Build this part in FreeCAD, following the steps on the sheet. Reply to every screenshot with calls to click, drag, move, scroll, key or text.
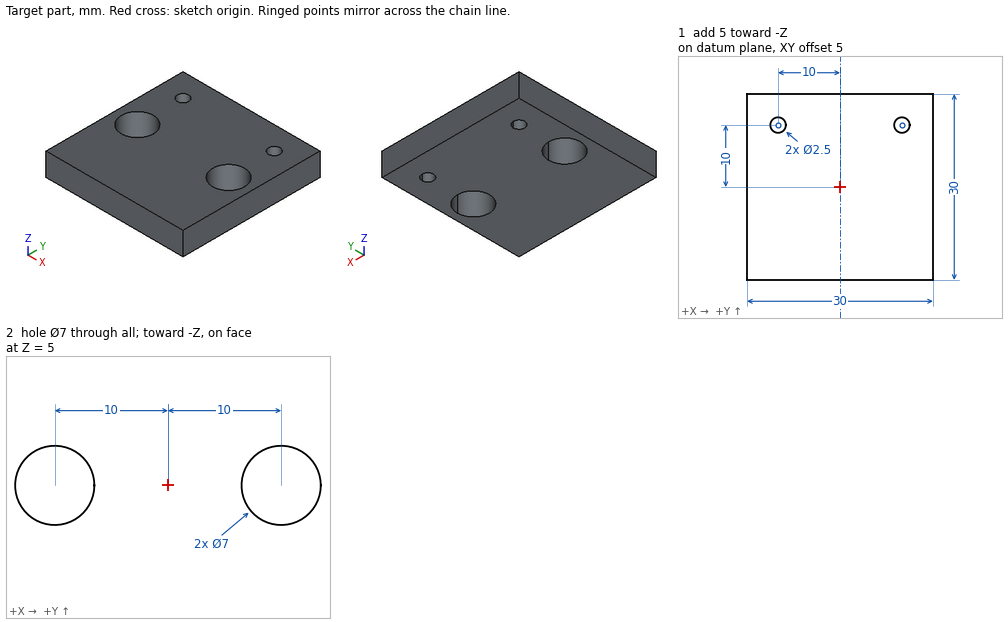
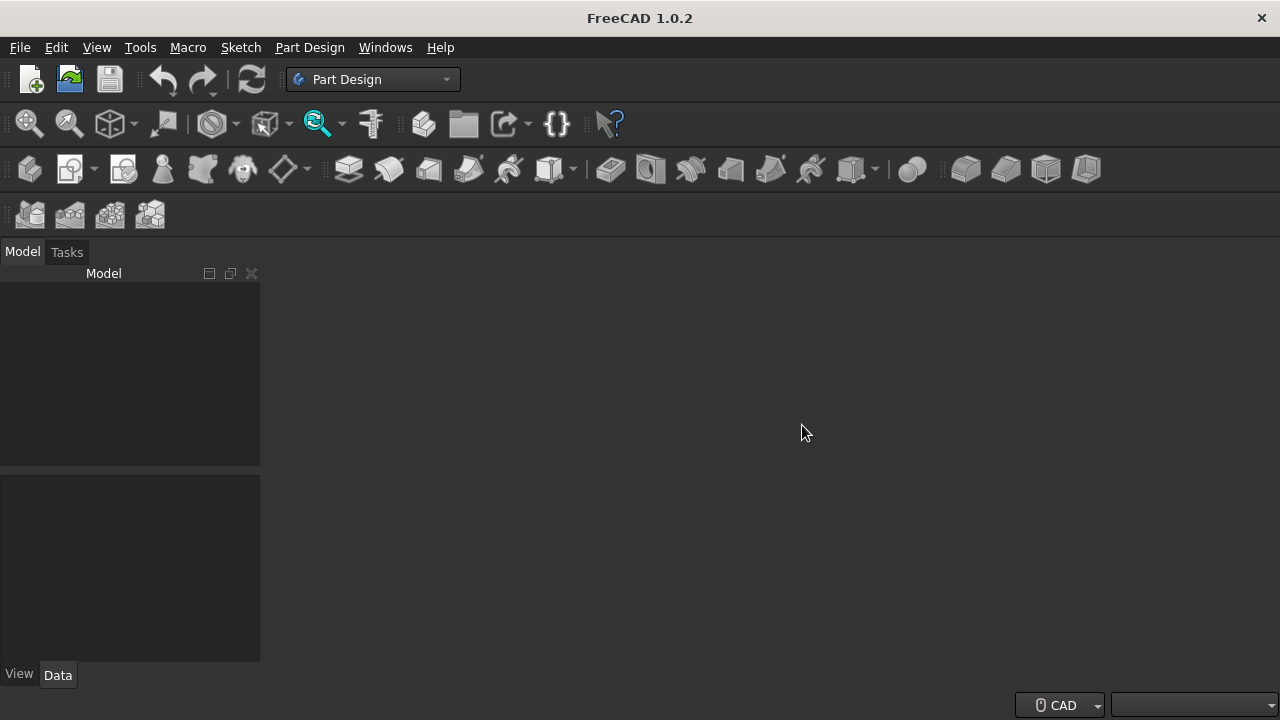
click(30, 80)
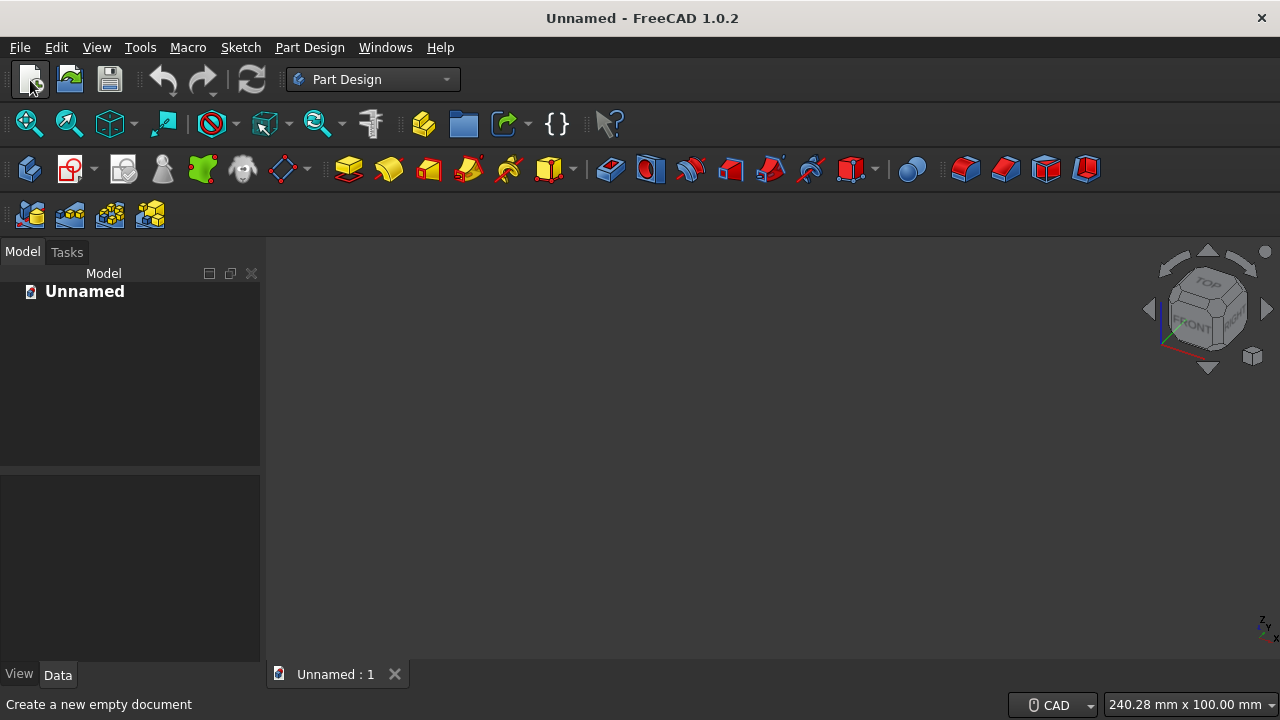
click(30, 170)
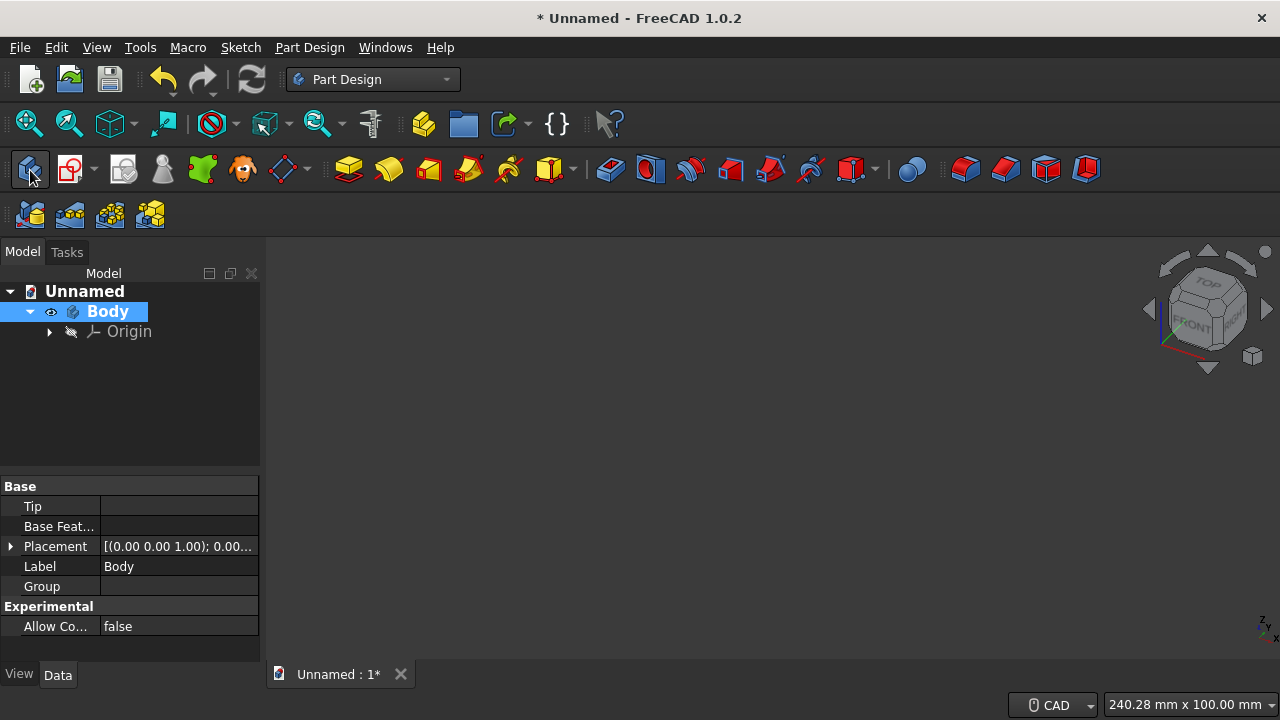
click(50, 332)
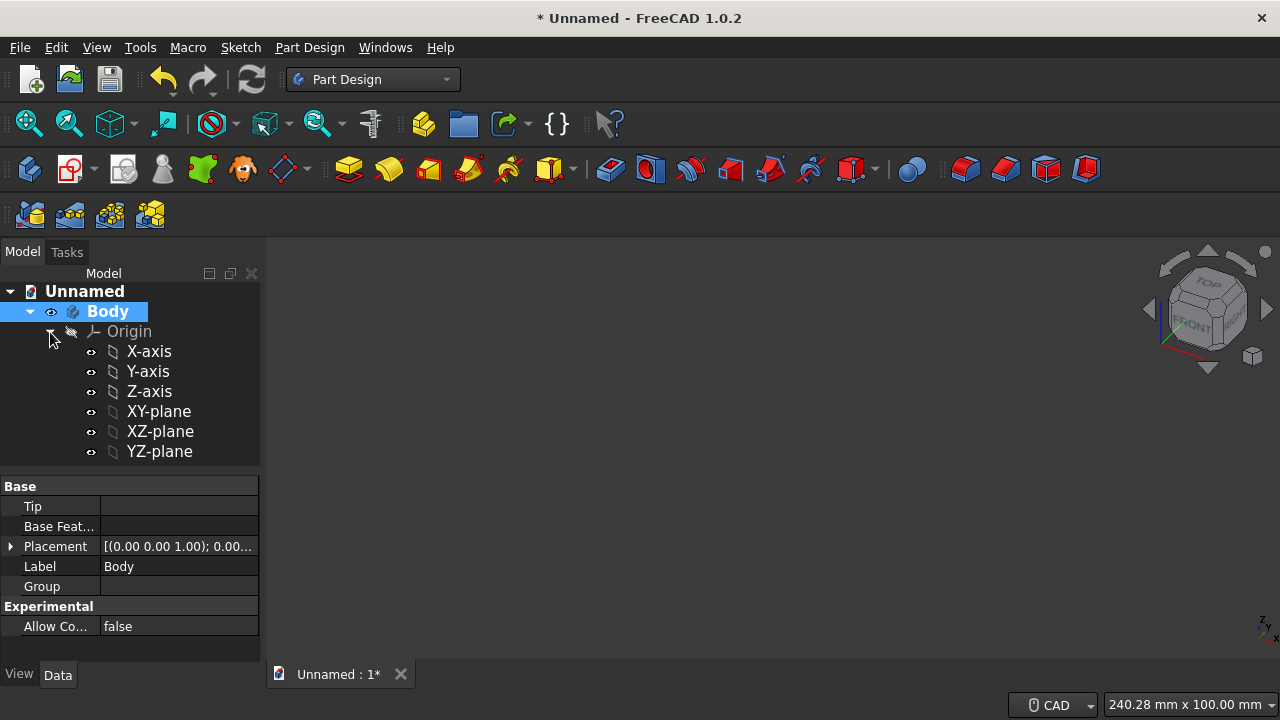
click(136, 412)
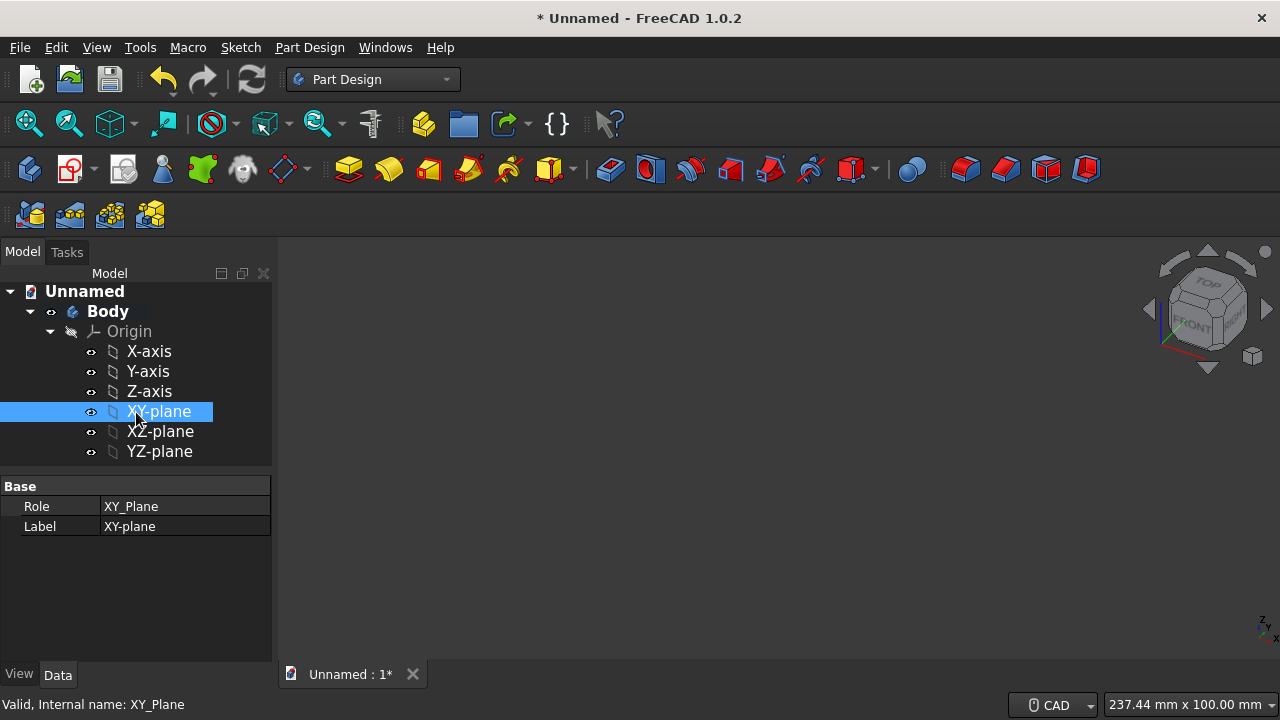
click(284, 170)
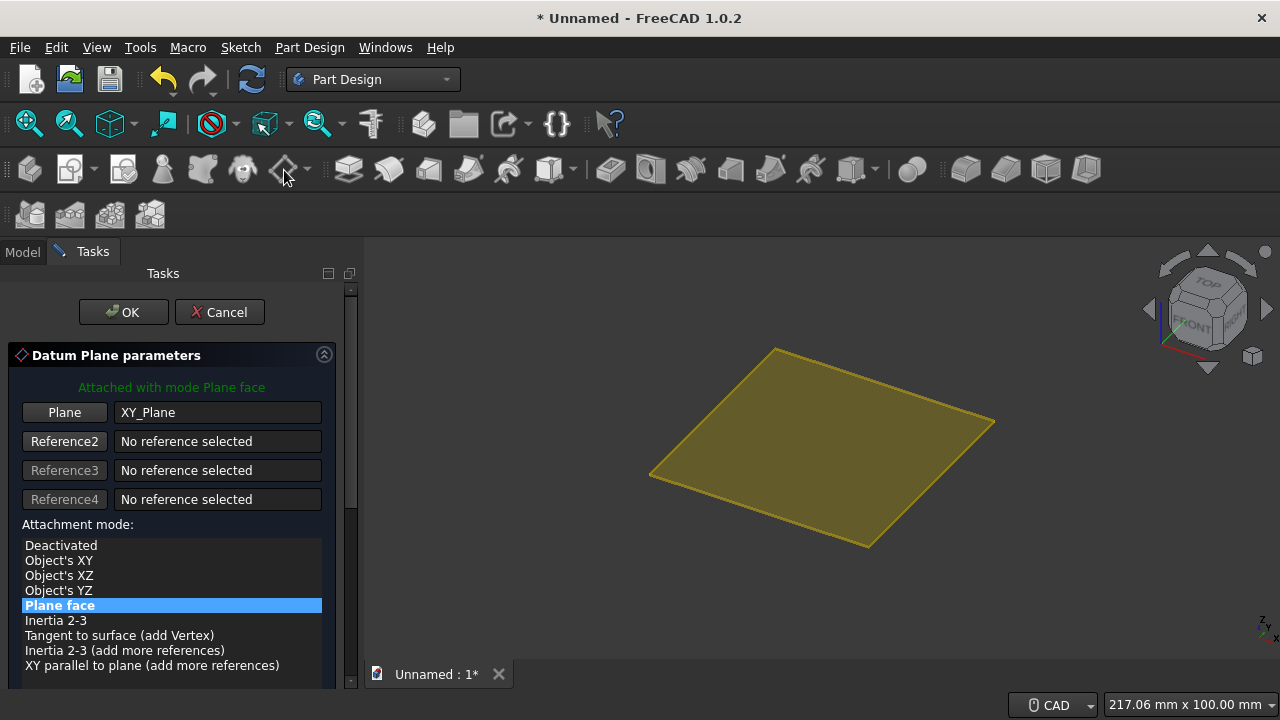
scroll(351, 486, down, 4)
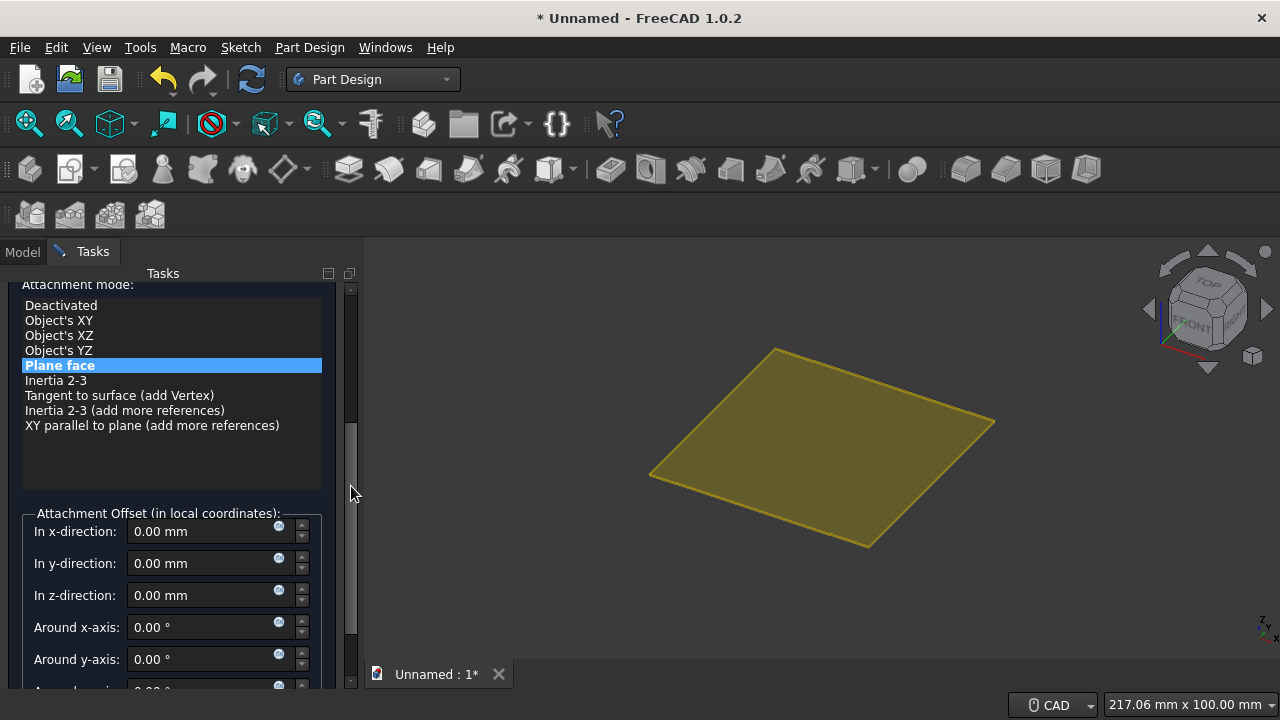
triple_click(210, 595)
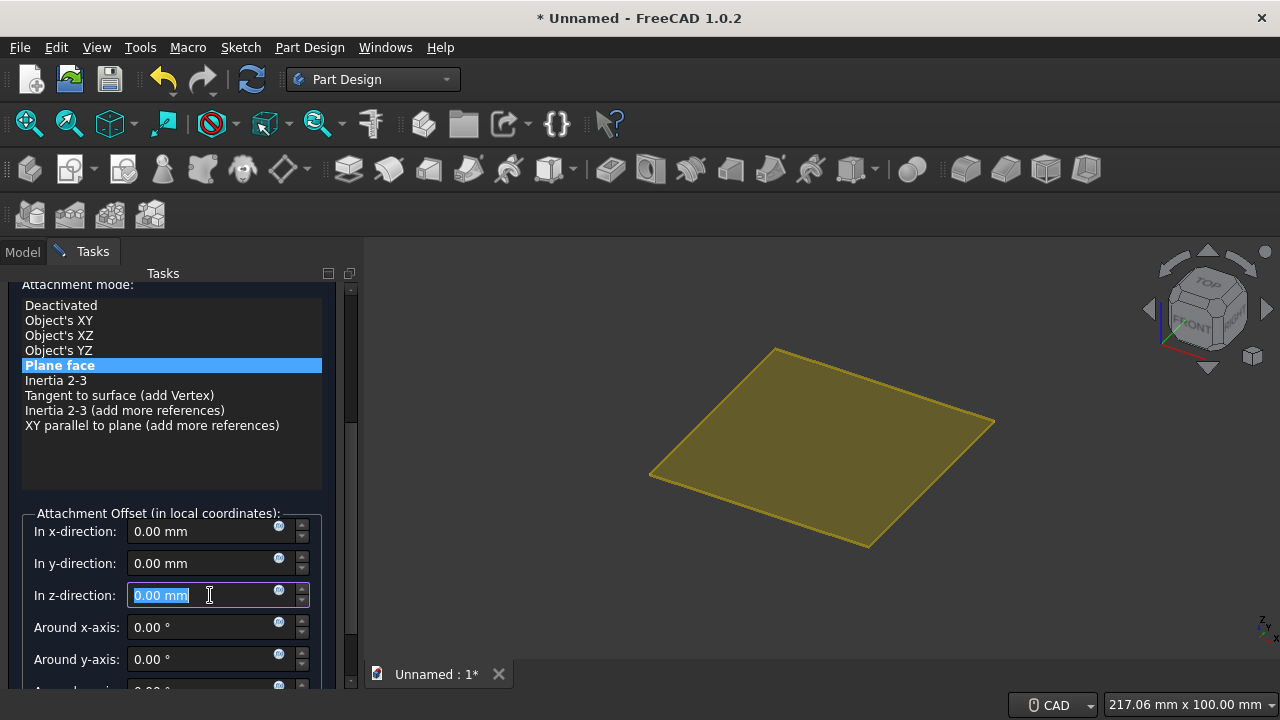
text(5)
key(Tab)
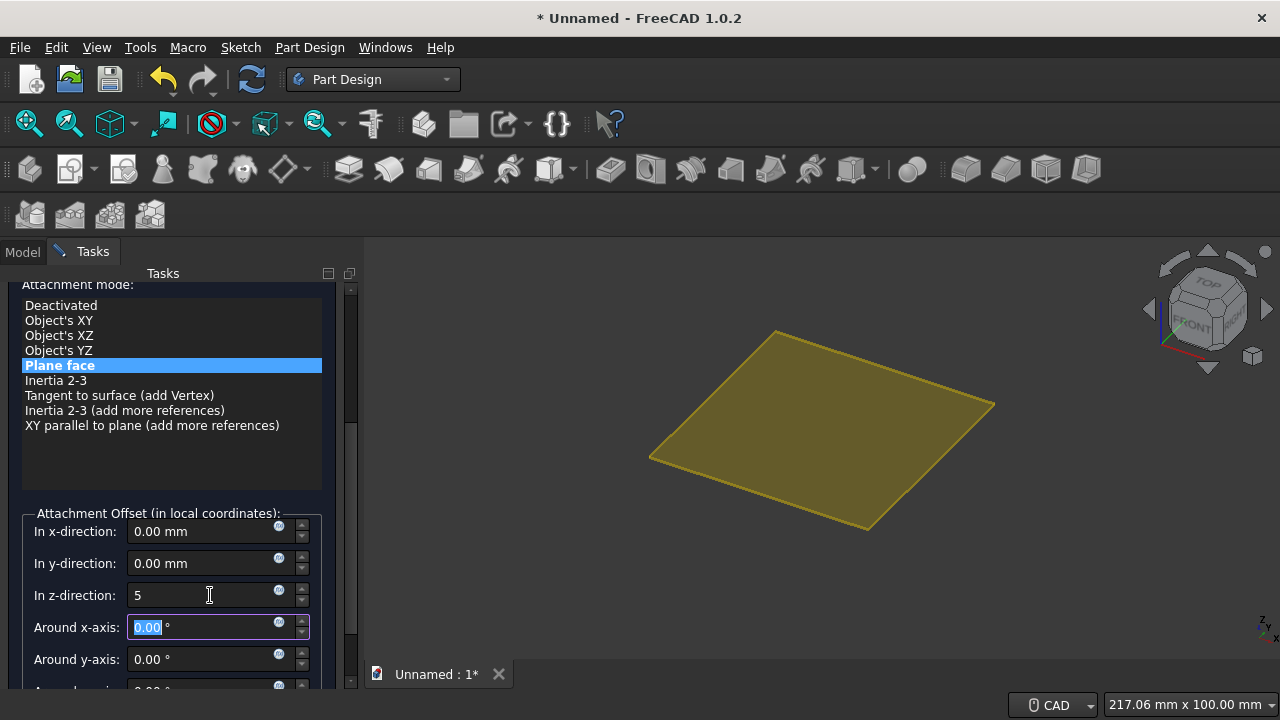
scroll(351, 486, up, 5)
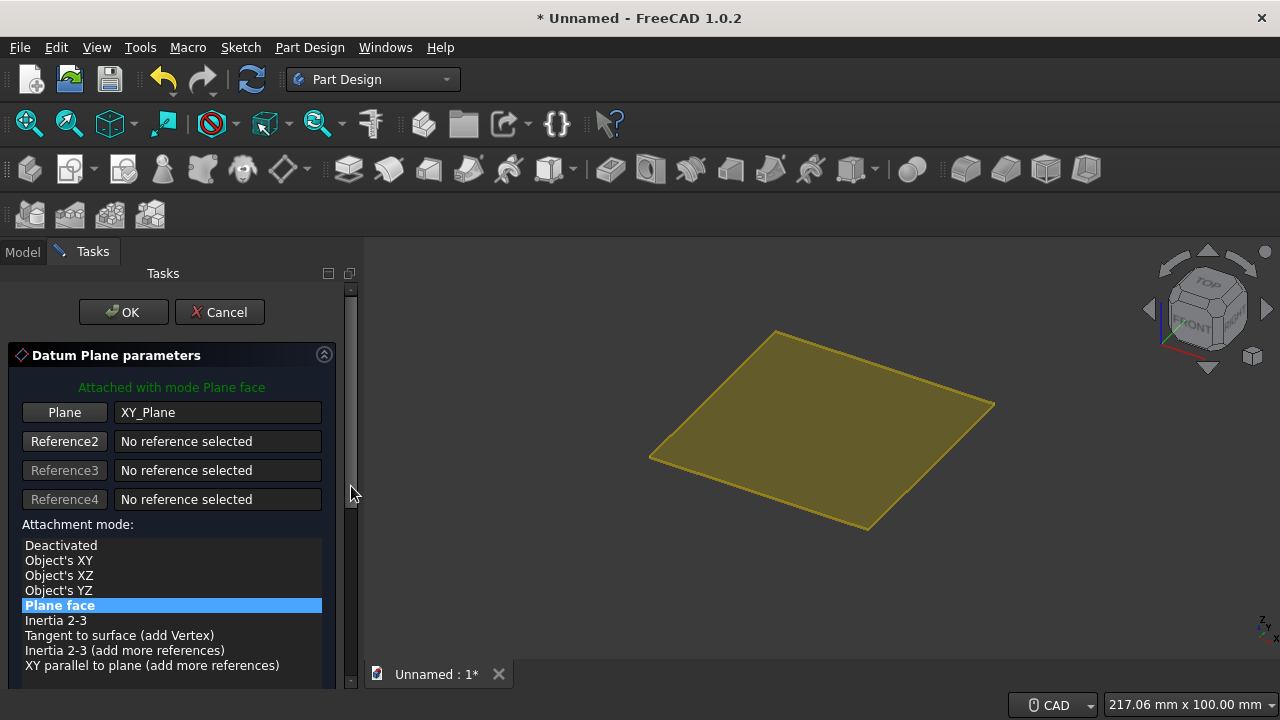
click(124, 312)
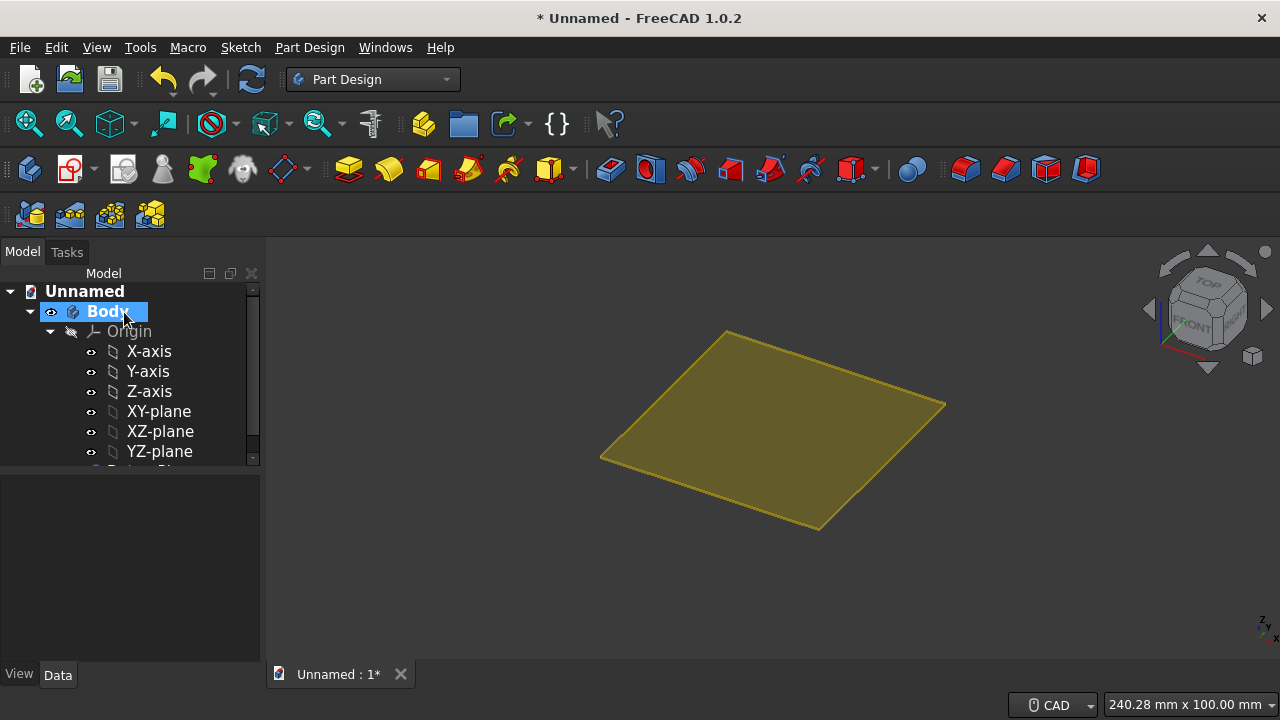
scroll(100, 367, down, 3)